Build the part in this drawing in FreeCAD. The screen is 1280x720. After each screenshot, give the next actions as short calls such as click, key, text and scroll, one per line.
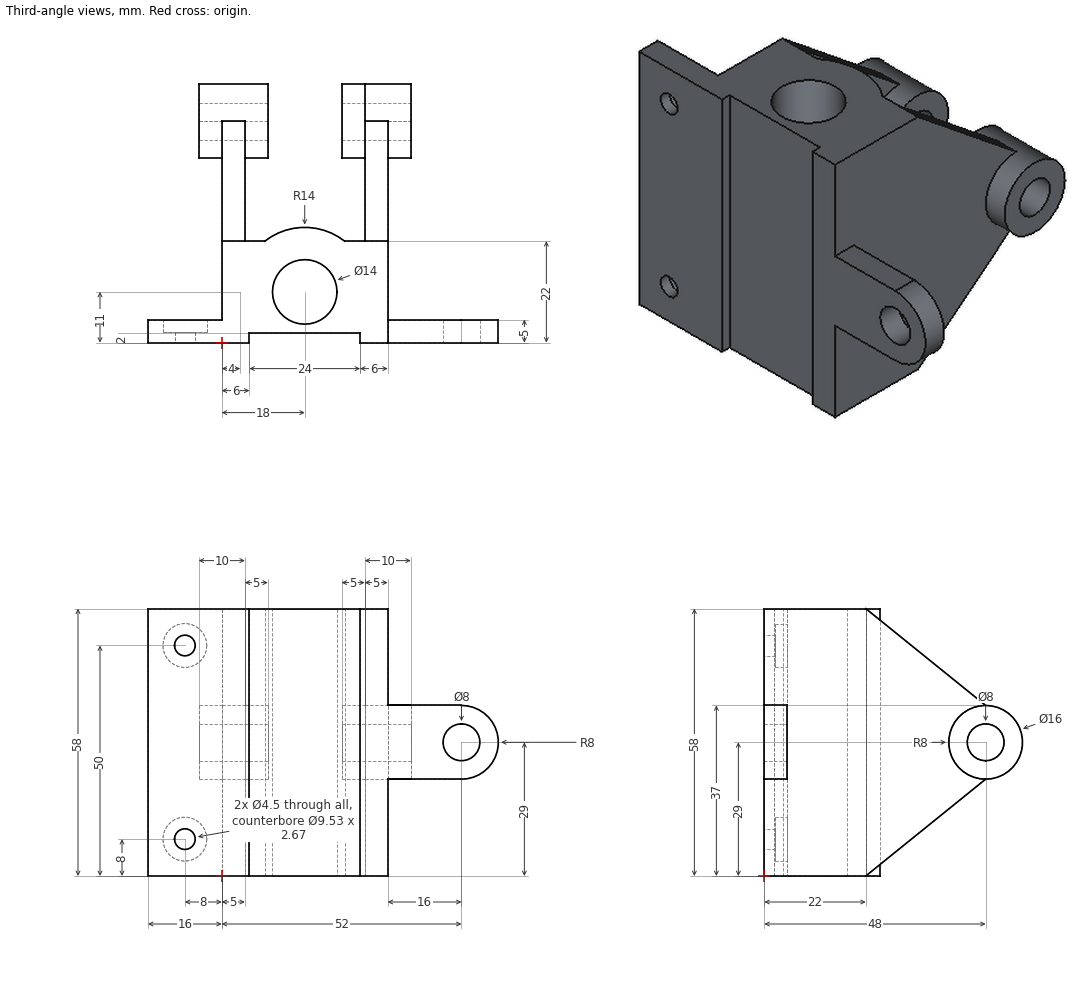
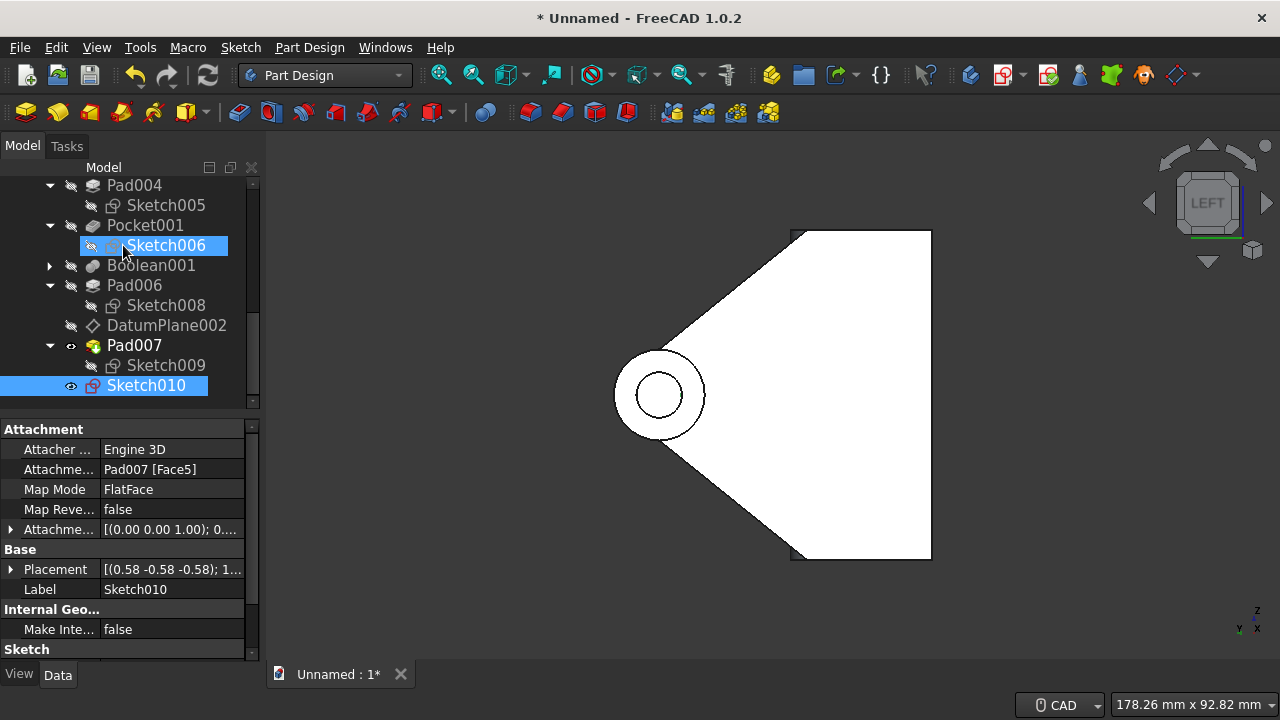
click(240, 112)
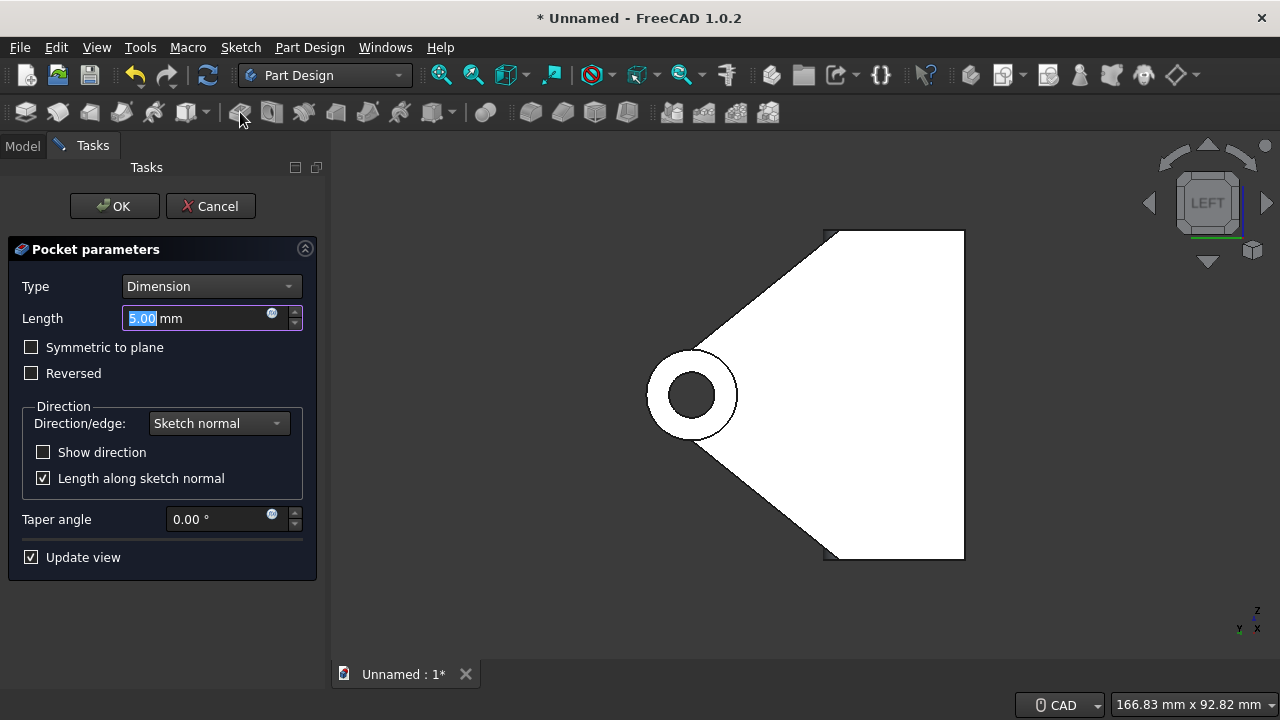
click(212, 286)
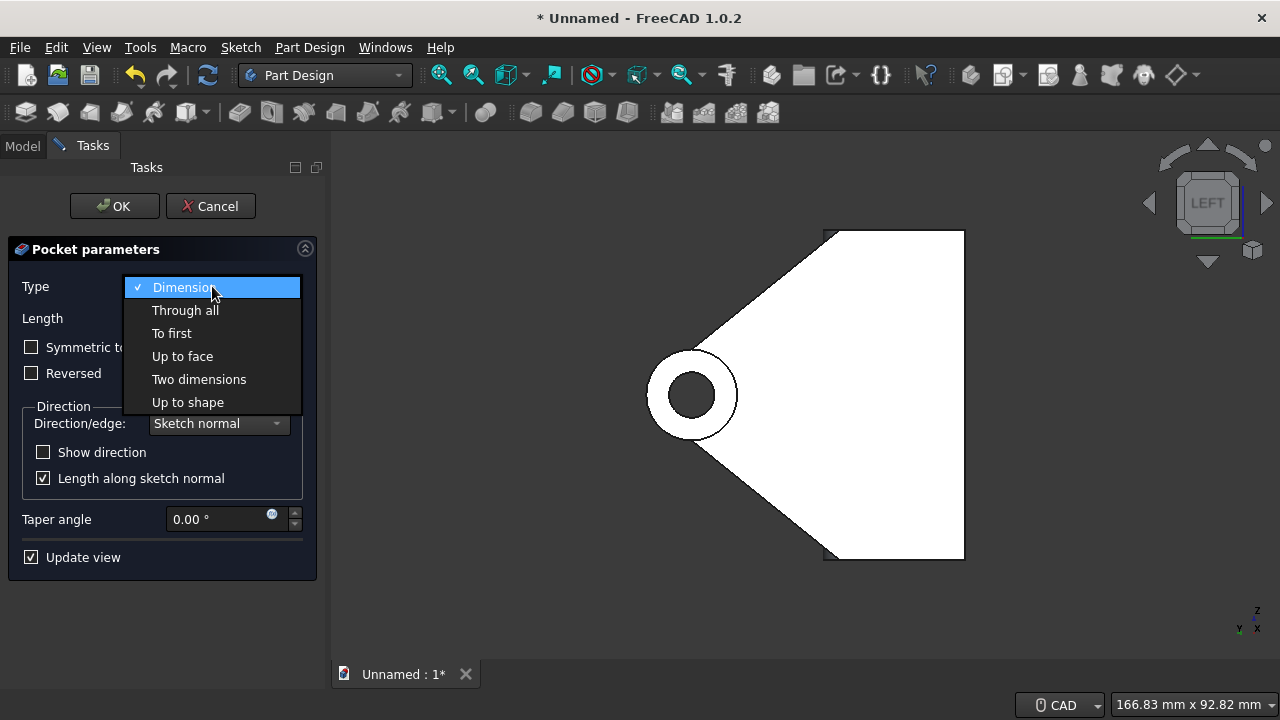
click(212, 310)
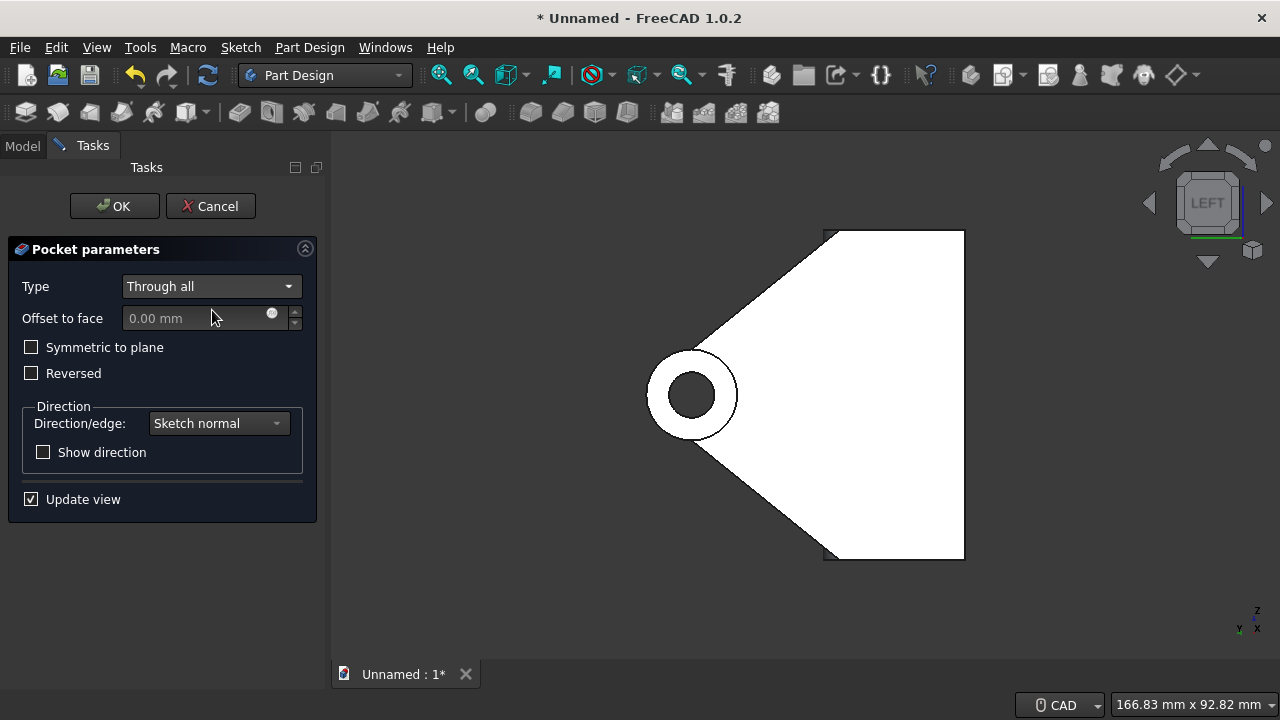
click(115, 206)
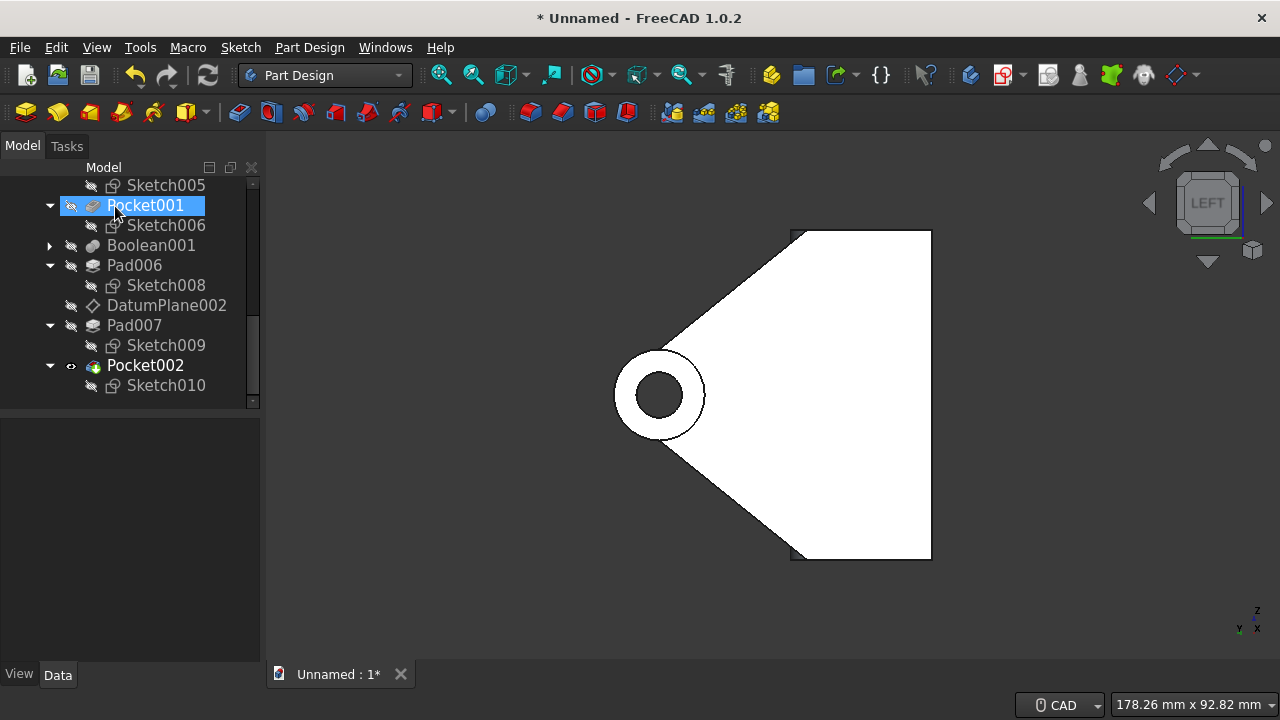
click(1004, 76)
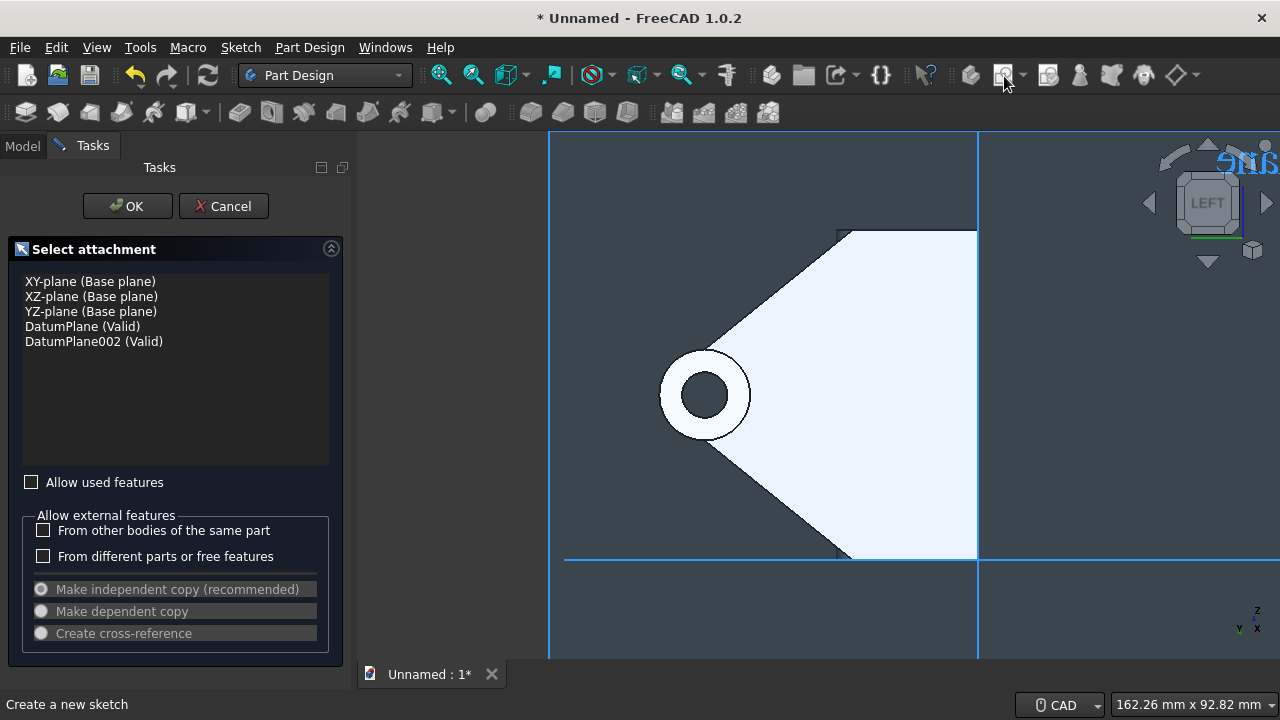
click(82, 296)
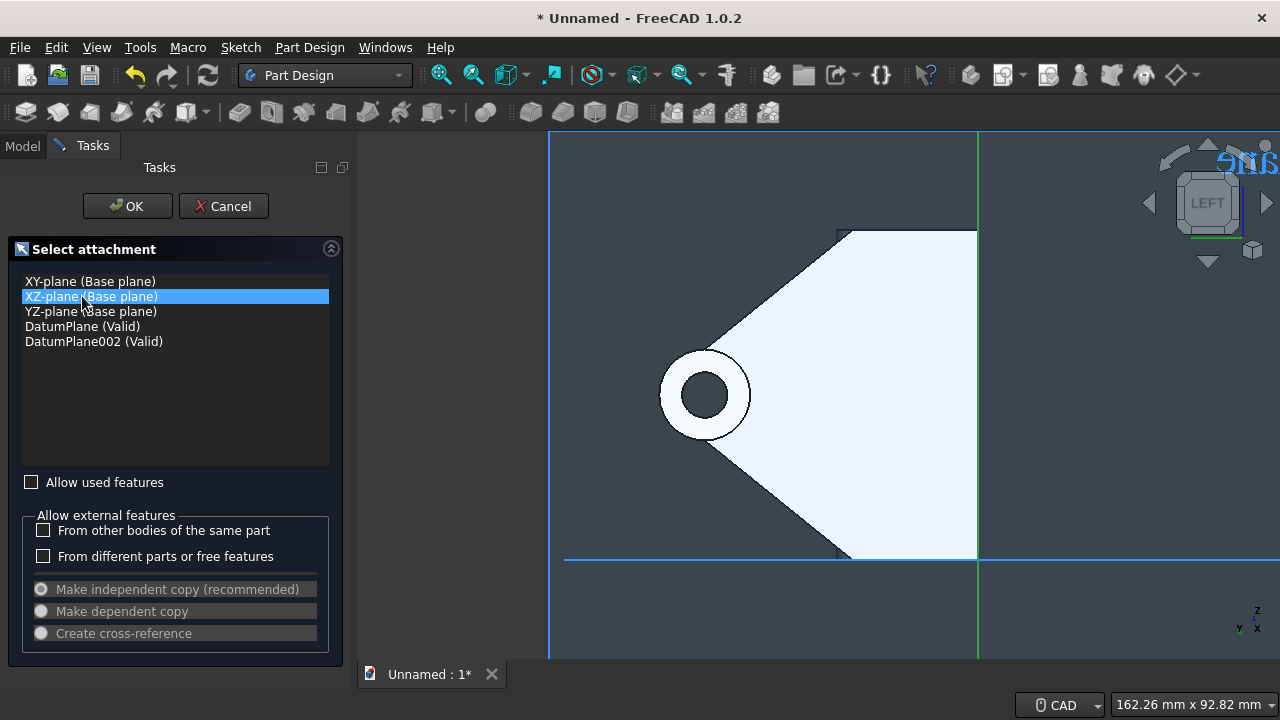
click(128, 206)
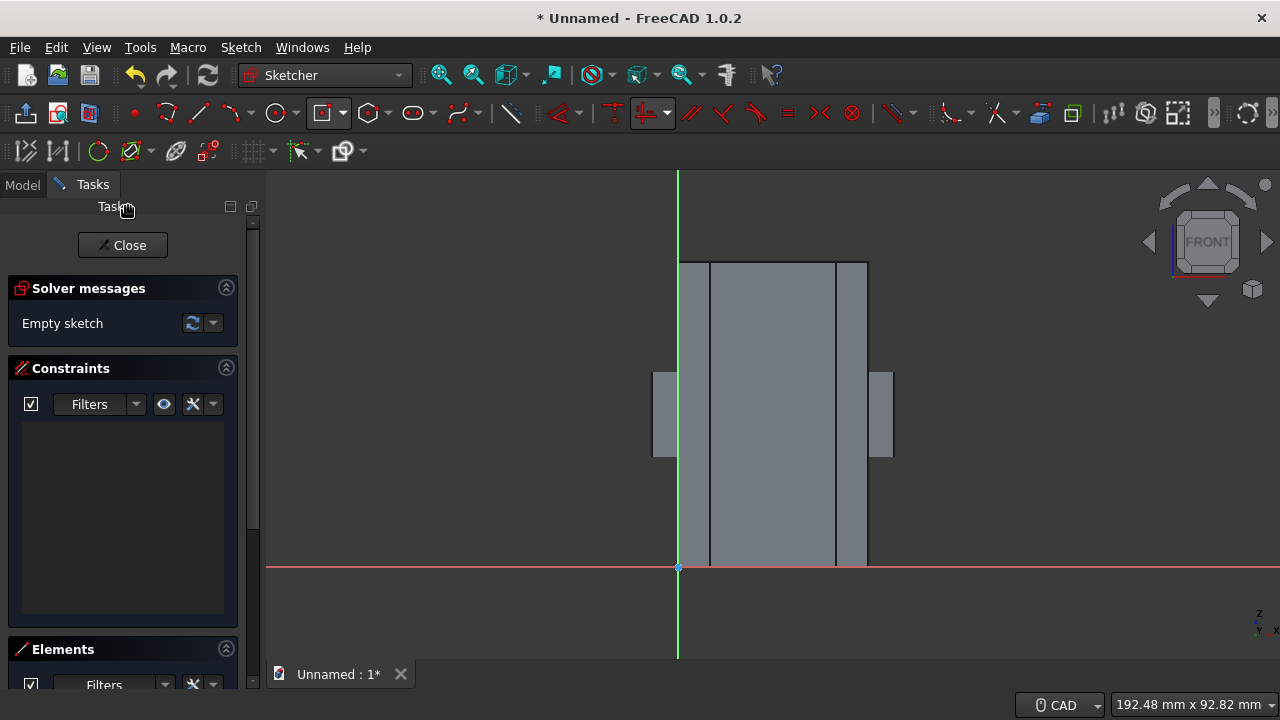
scroll(1029, 415, up, 6)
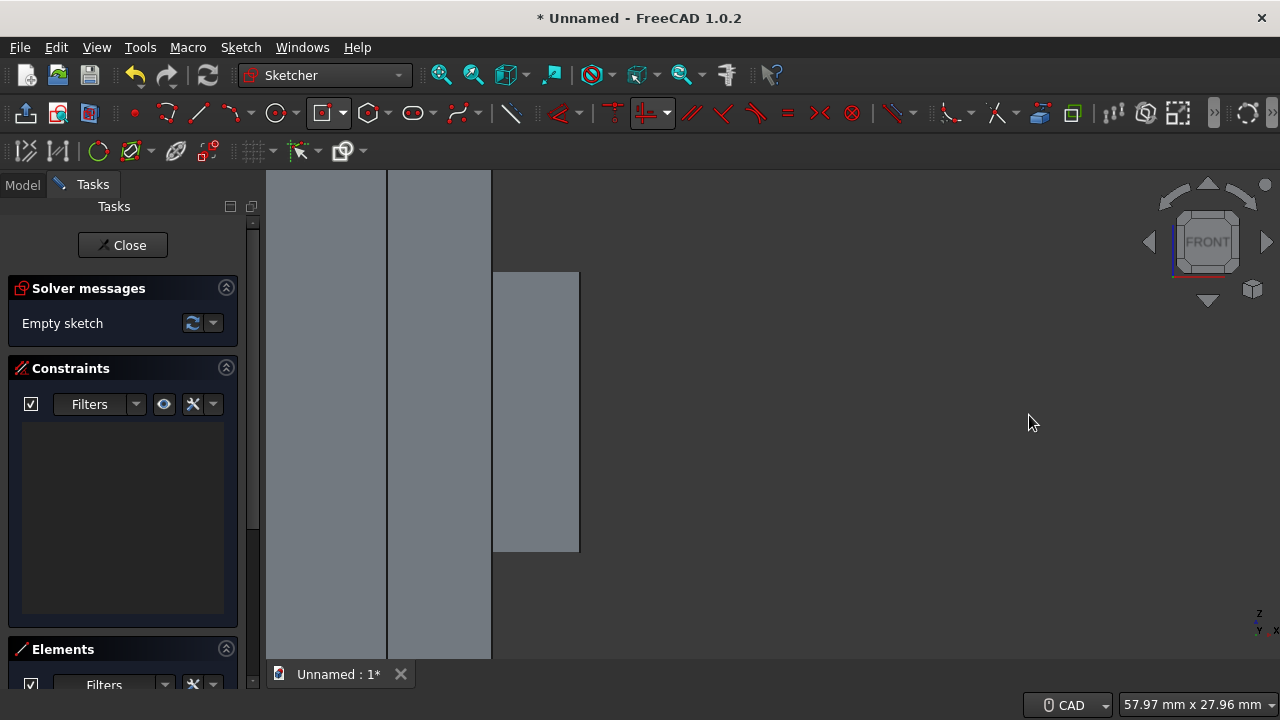
key(g)
key(m)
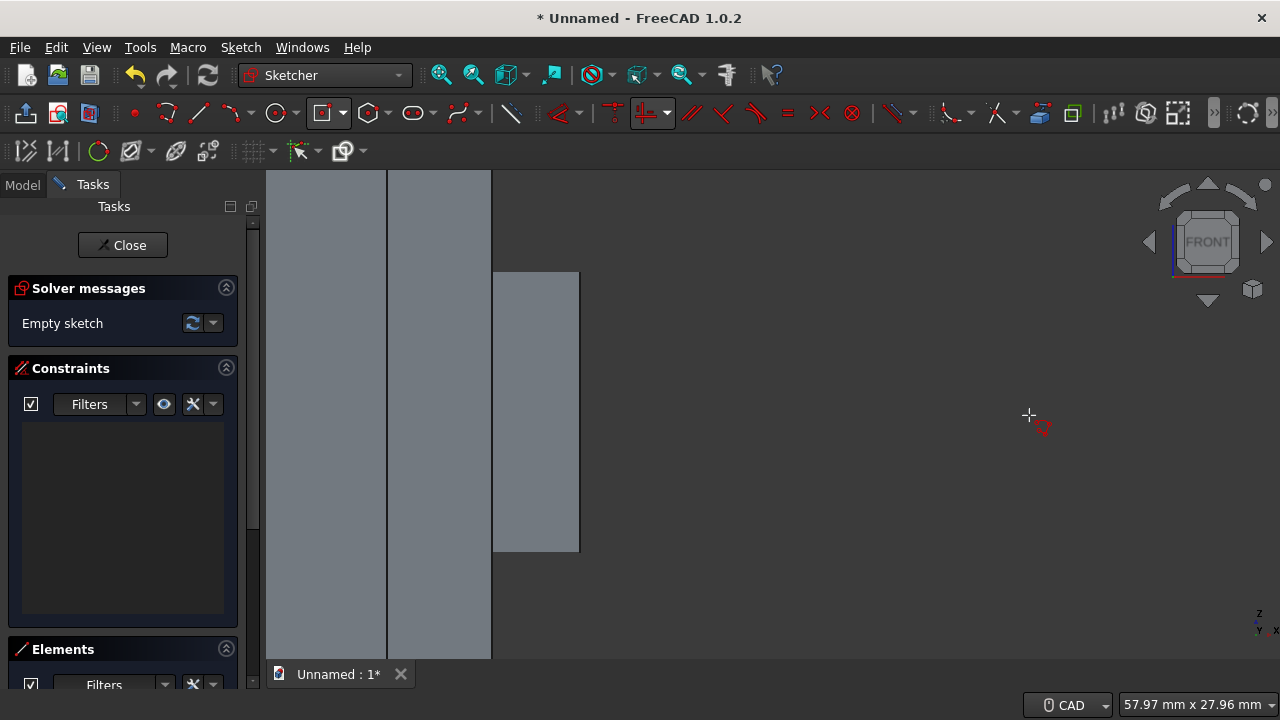
click(772, 552)
click(492, 552)
click(492, 272)
click(772, 272)
right_click(772, 272)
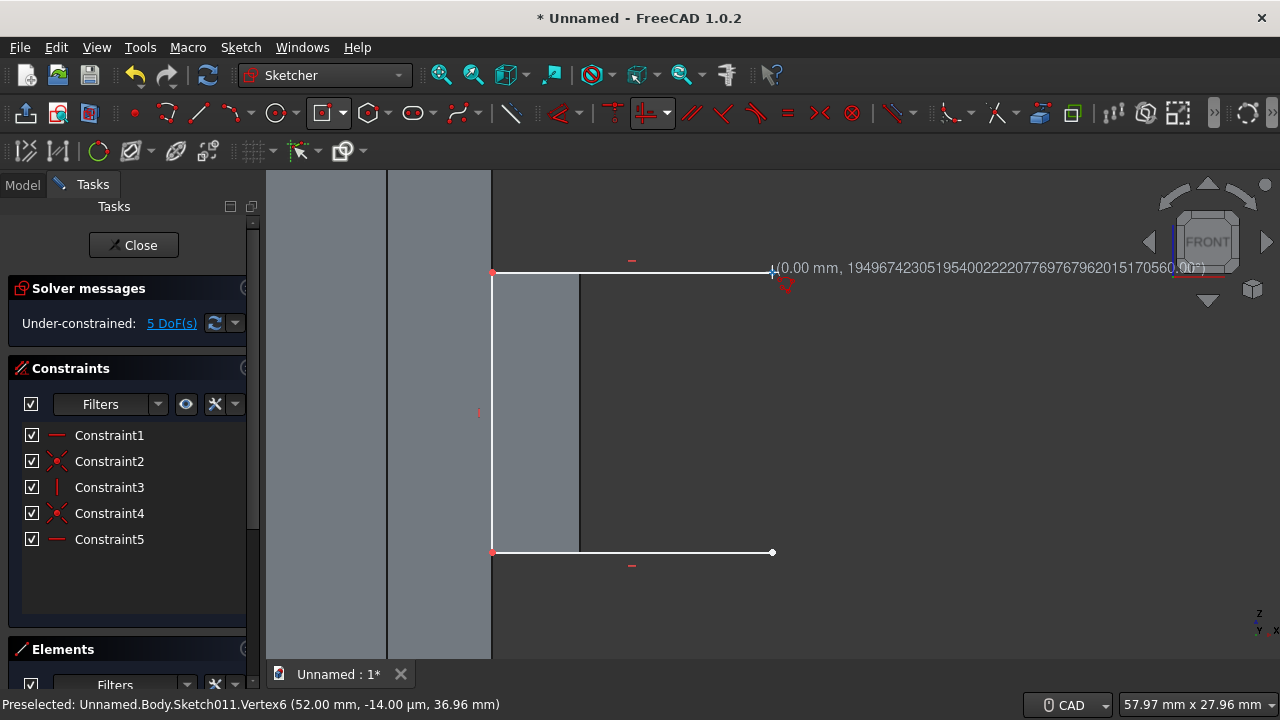
key(g)
key(3)
key(a)